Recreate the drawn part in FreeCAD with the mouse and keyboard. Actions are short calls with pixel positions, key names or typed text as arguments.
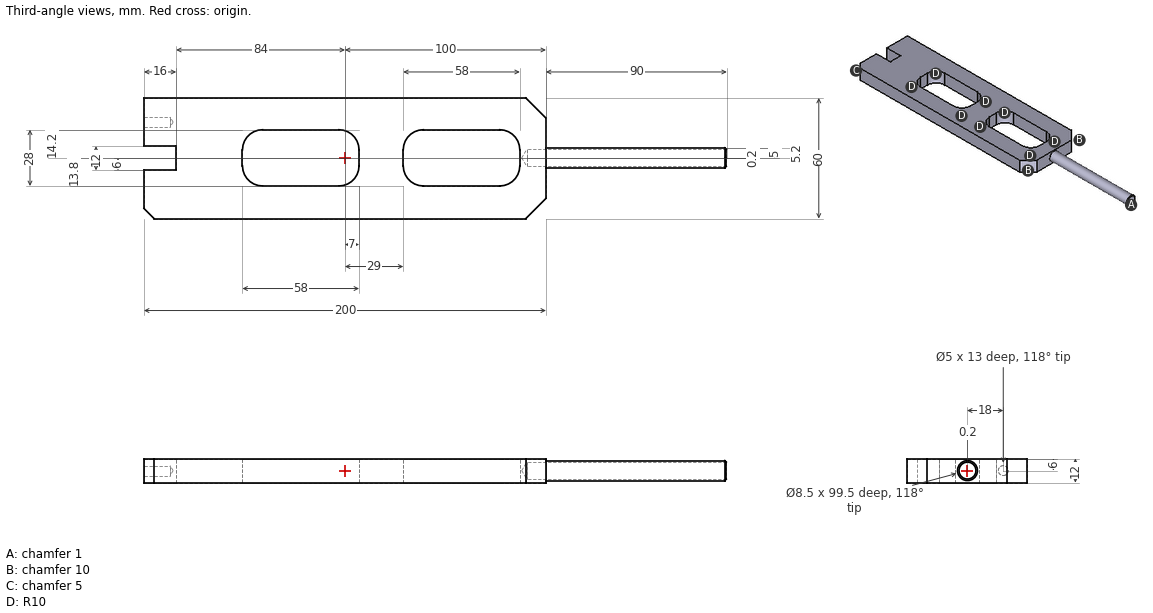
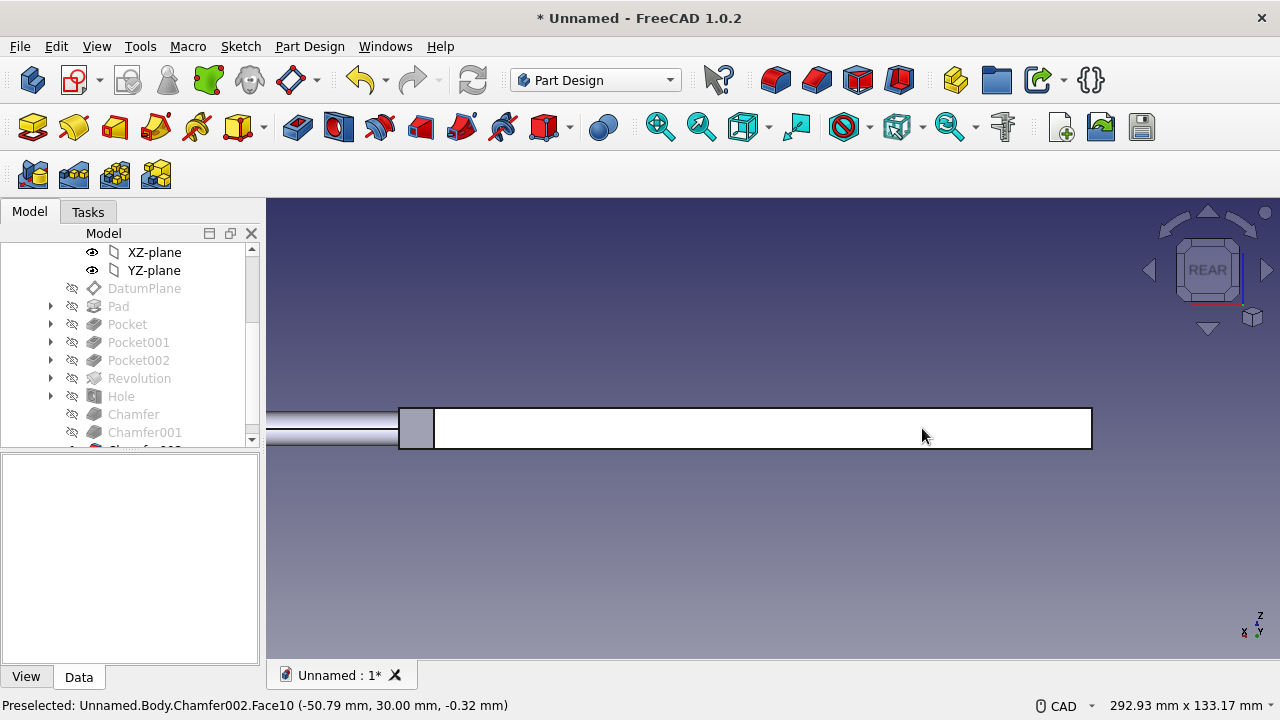
click(661, 128)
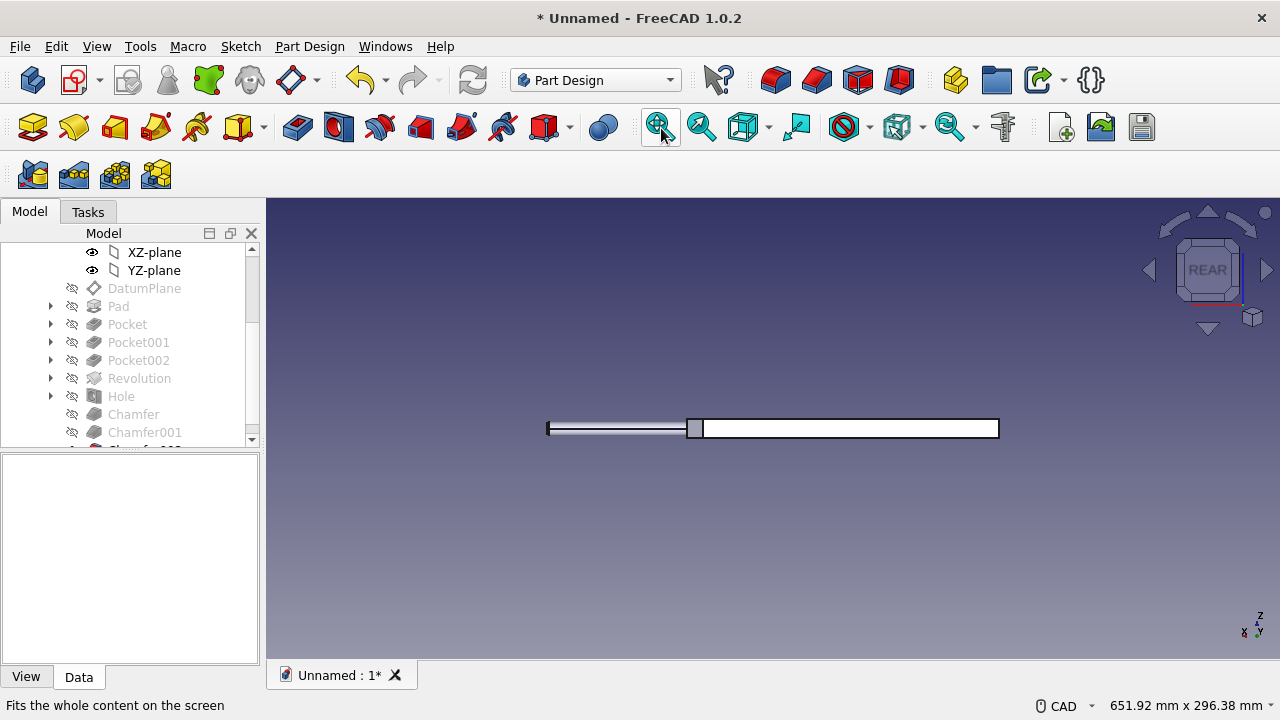
key(6)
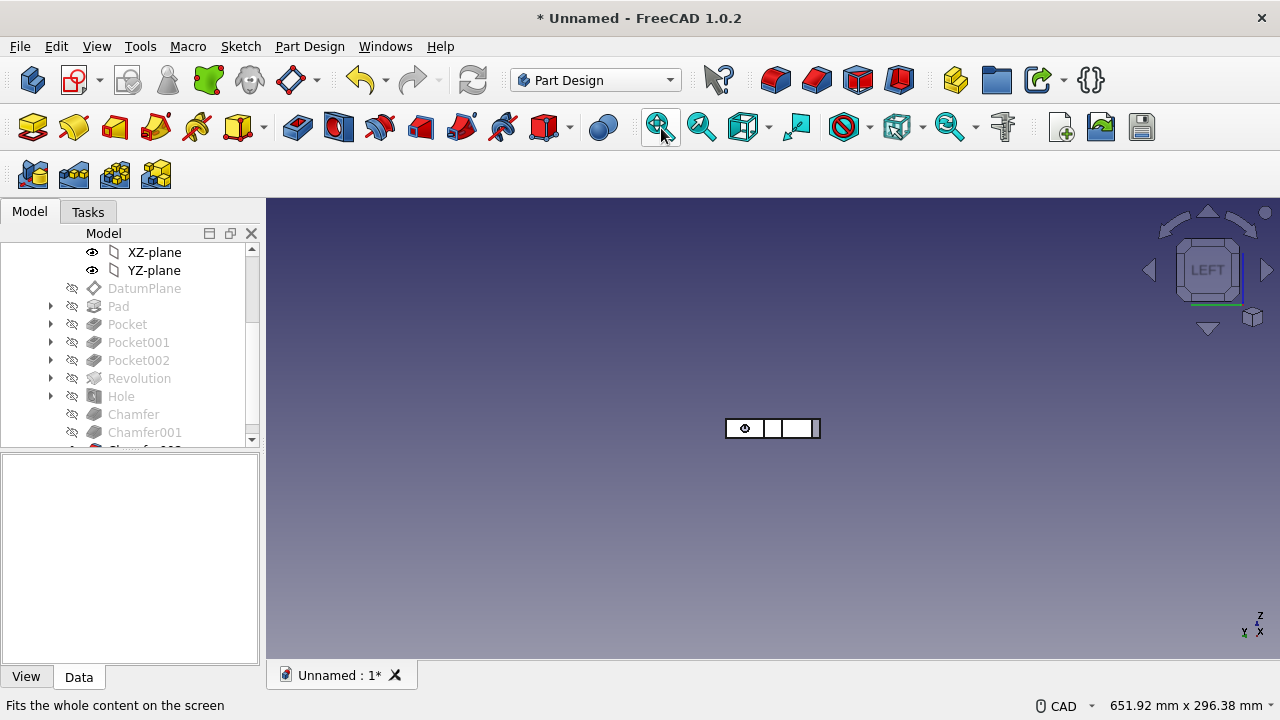
click(661, 128)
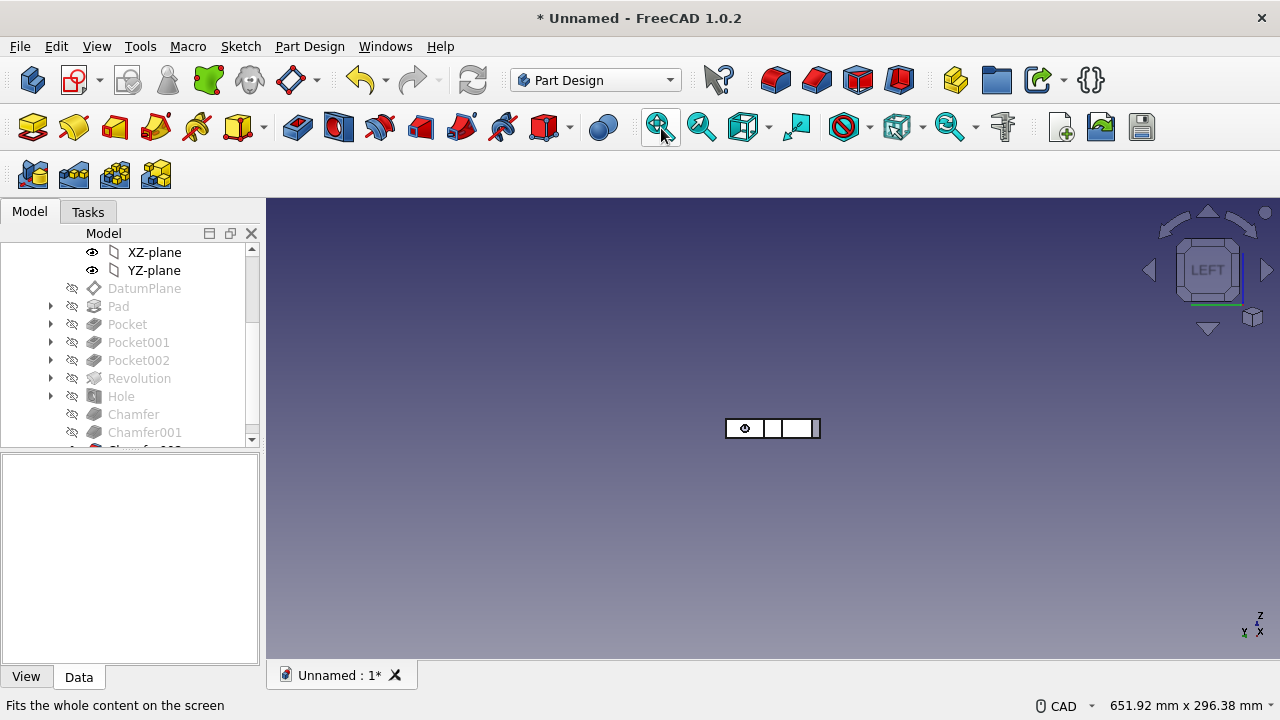
scroll(794, 427, up, 4)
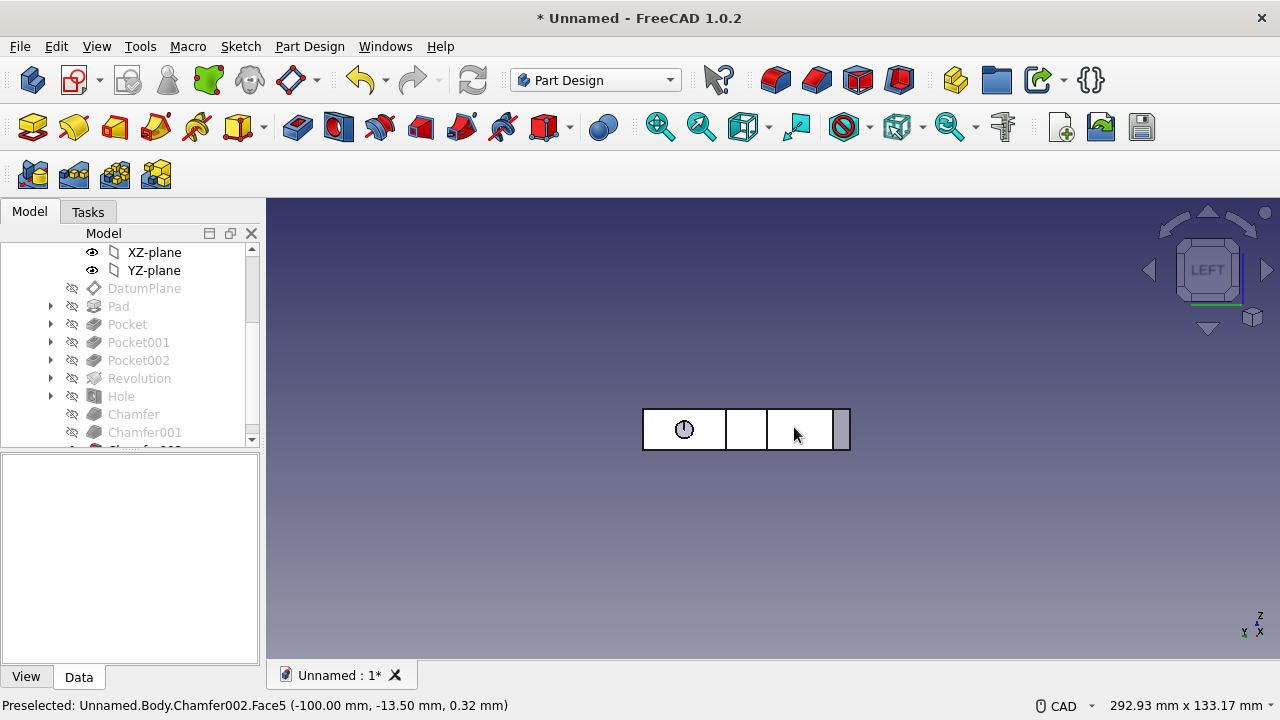
key(v)
key(f)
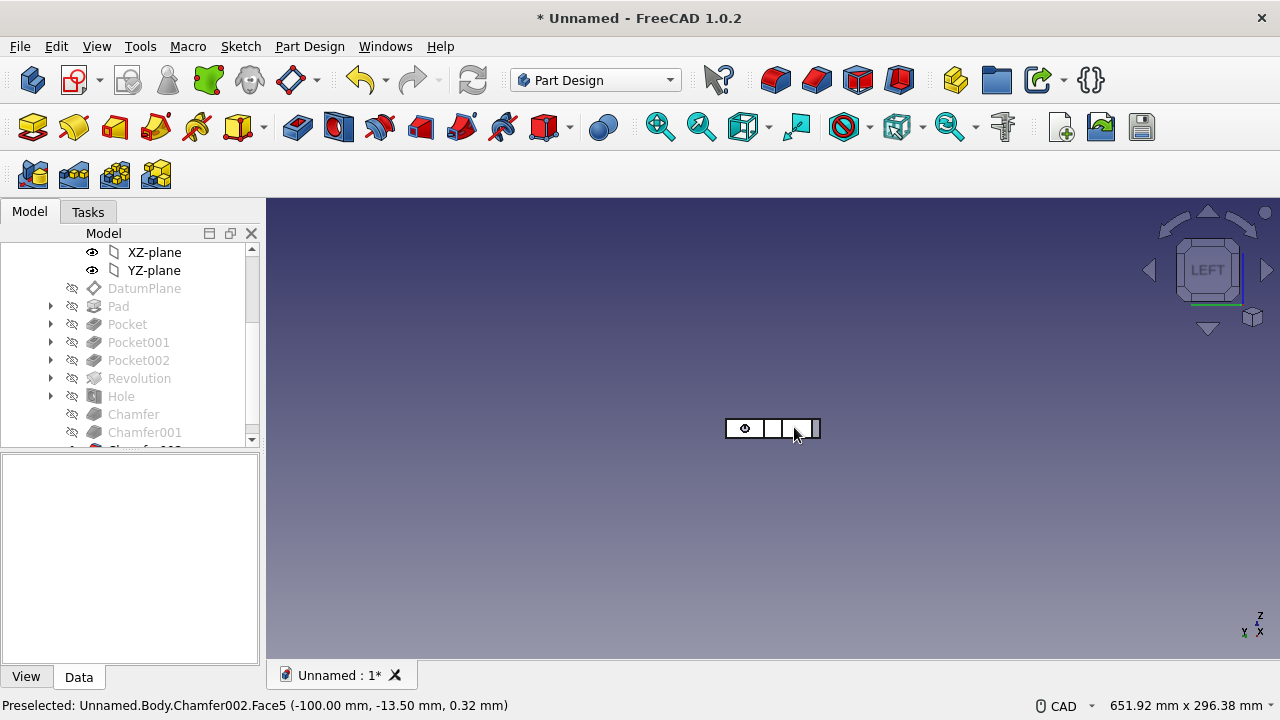
key(v)
key(3)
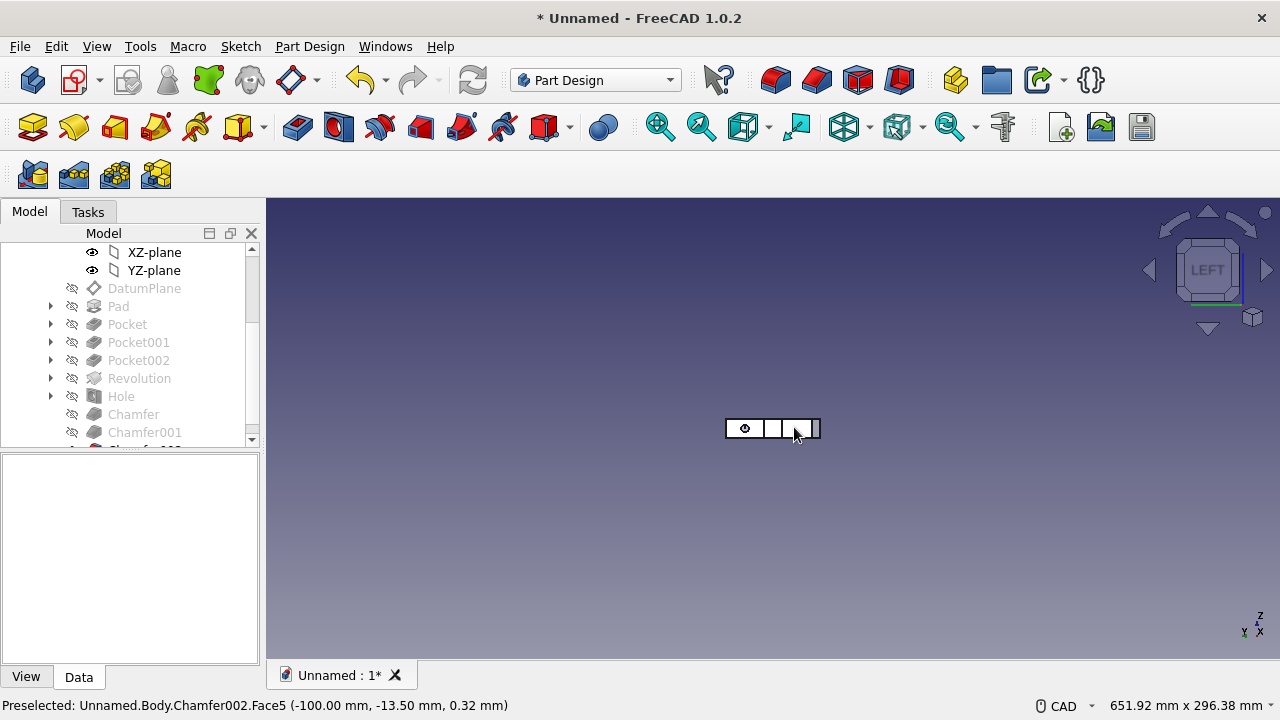
key(0)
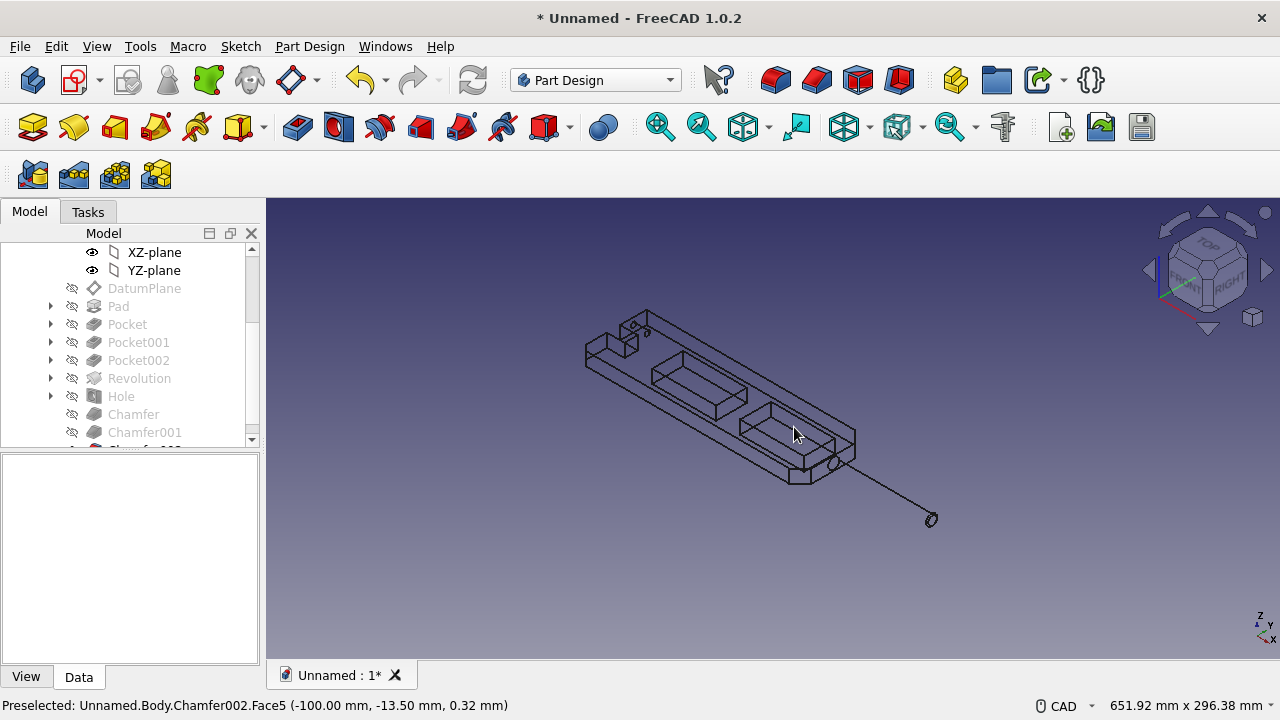
click(652, 375)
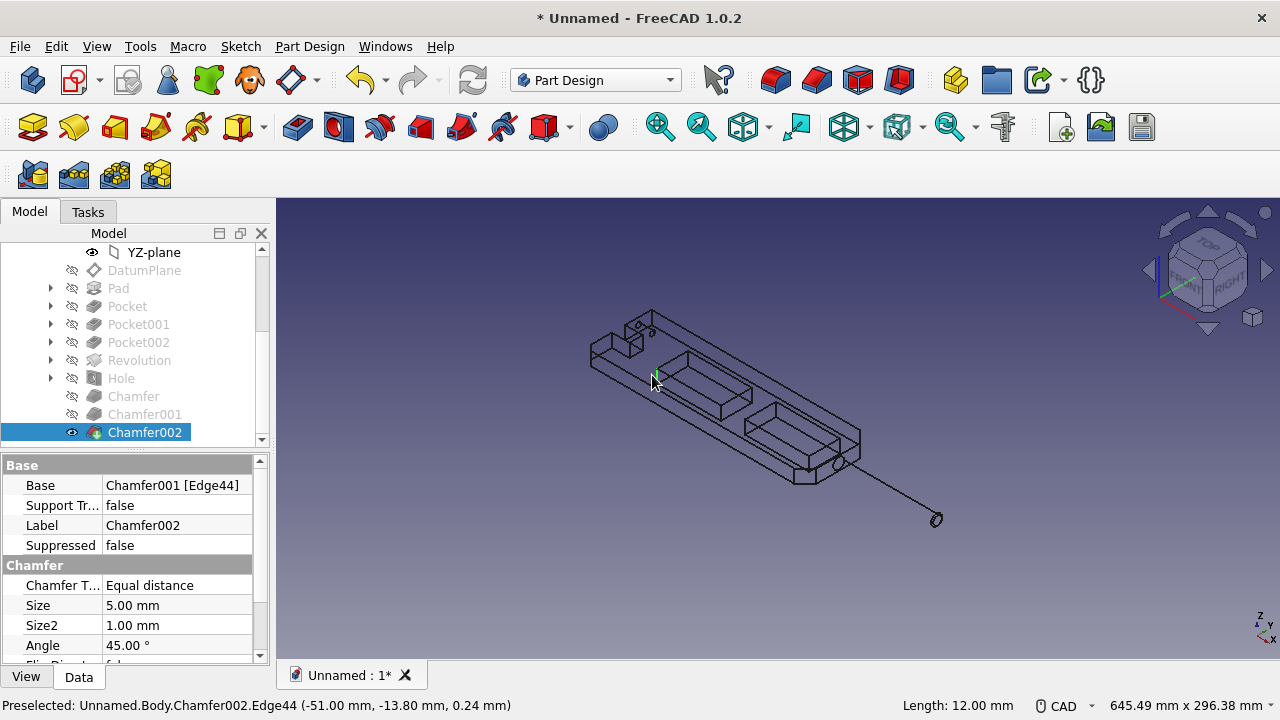
click(688, 358, ctrl)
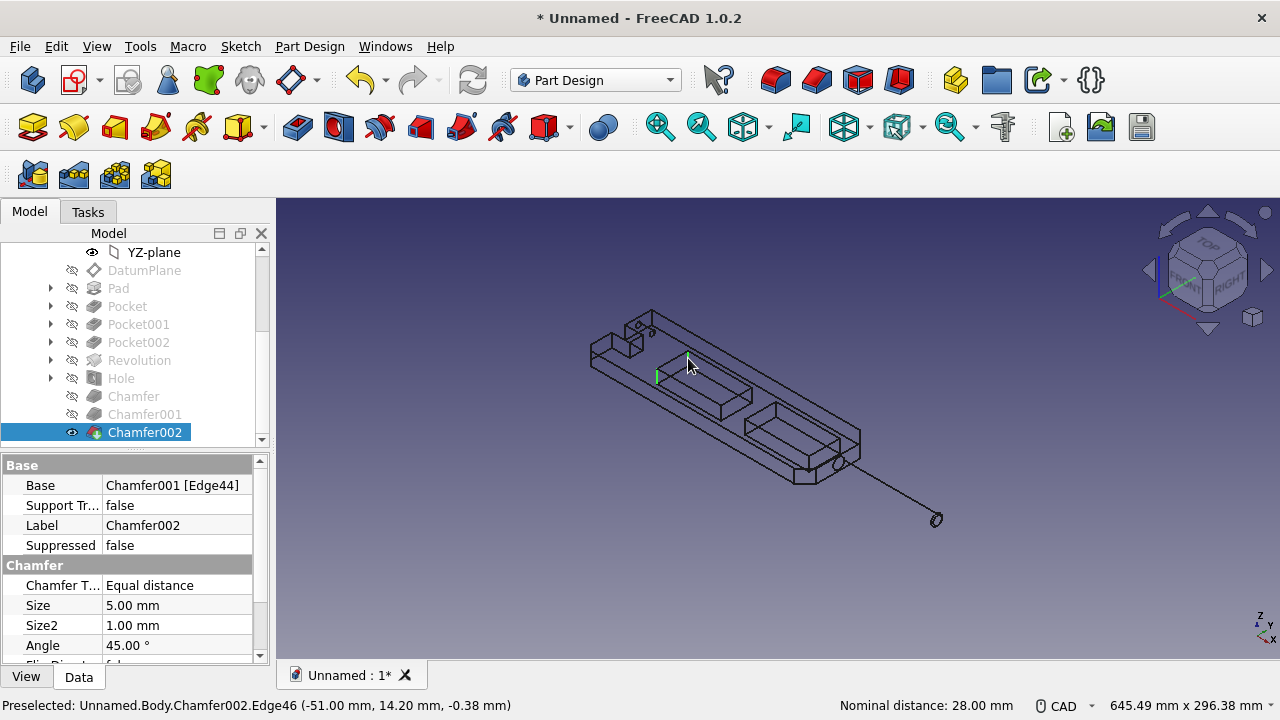
click(752, 394, ctrl)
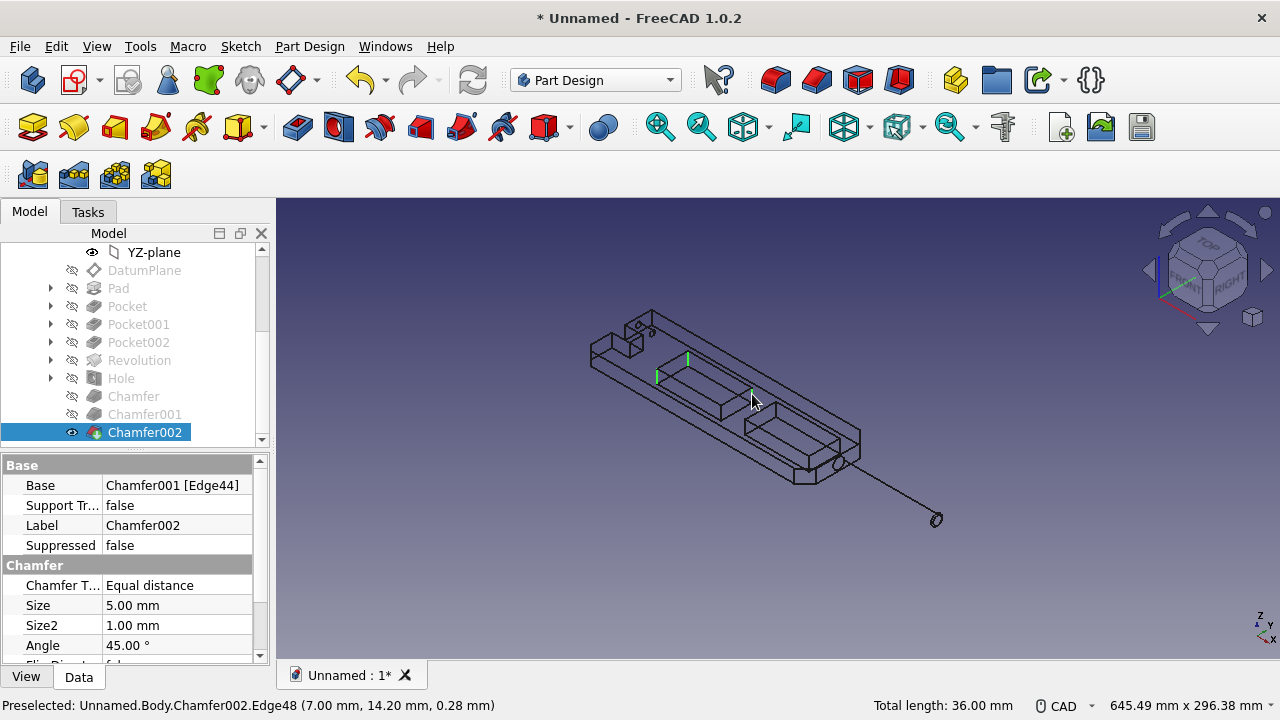
click(721, 412, ctrl)